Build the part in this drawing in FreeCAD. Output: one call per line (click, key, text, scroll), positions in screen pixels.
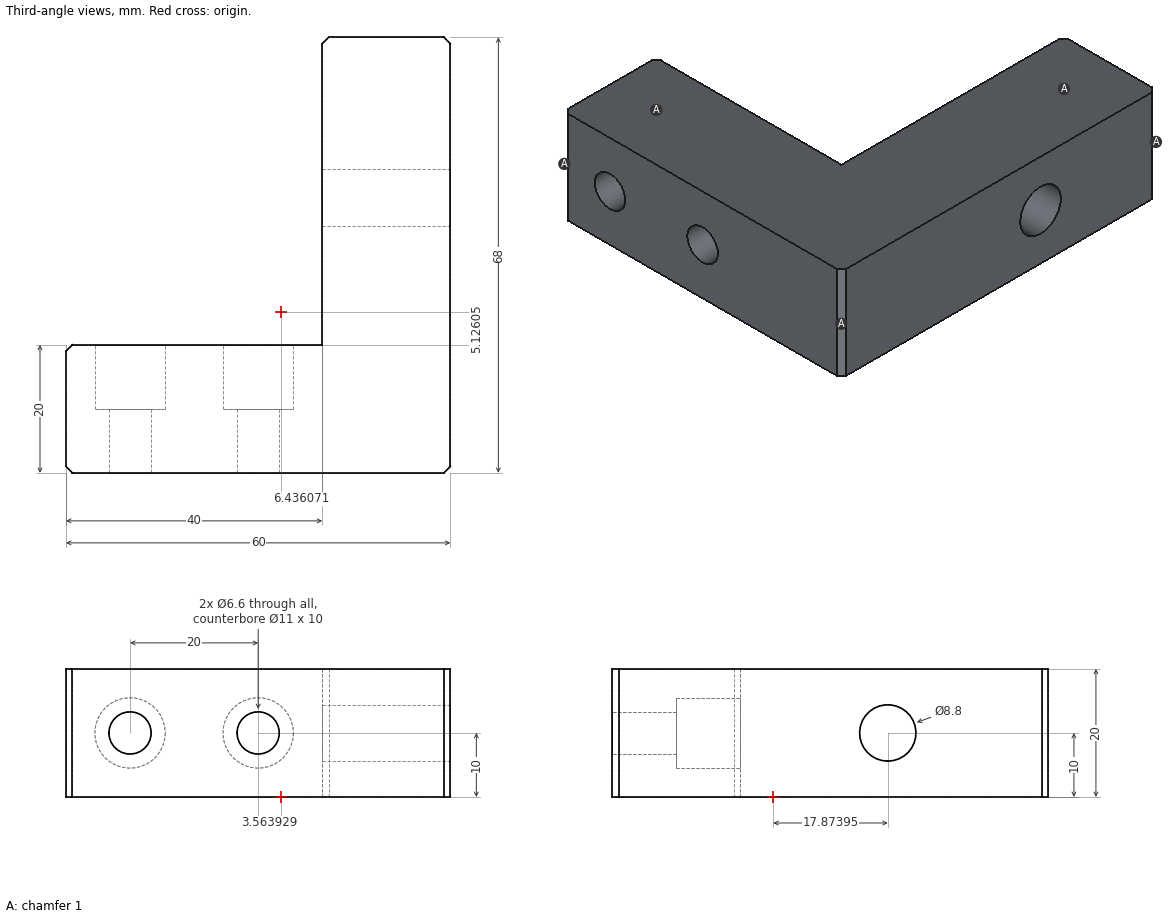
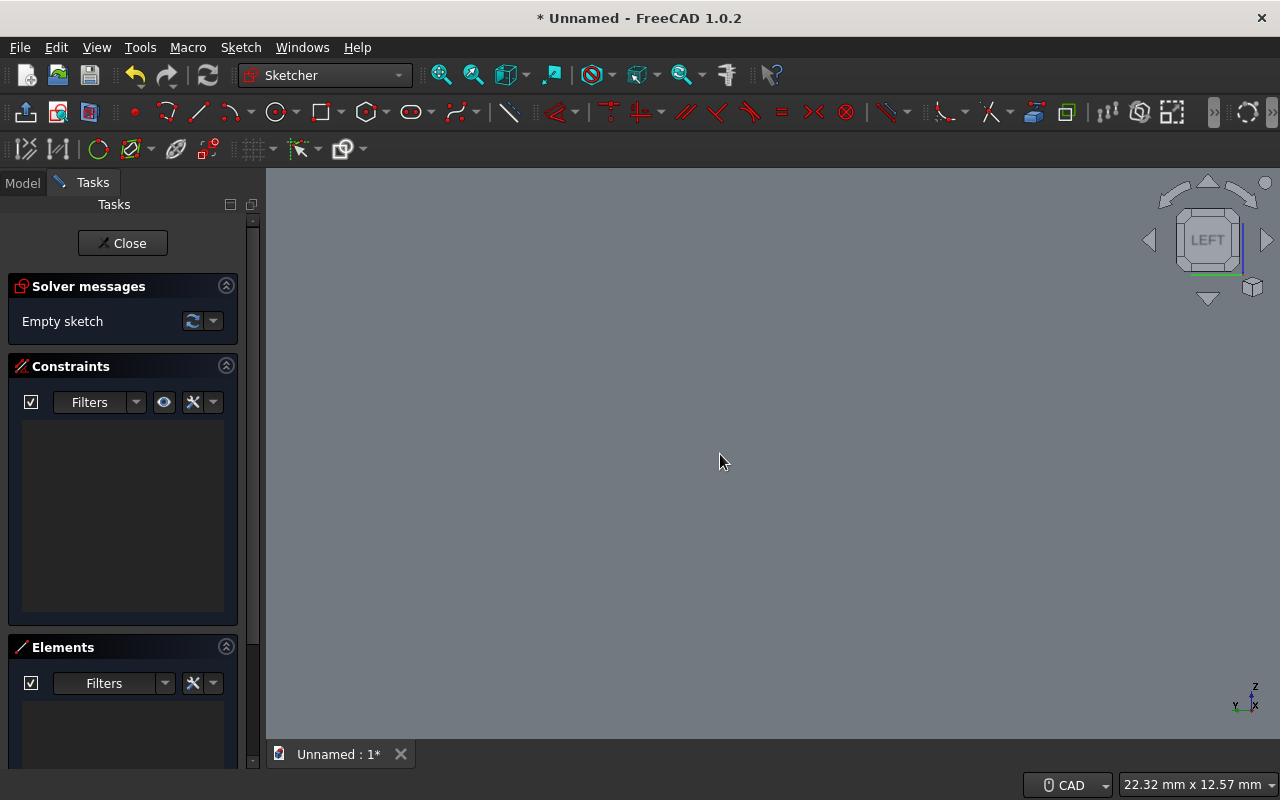
click(276, 112)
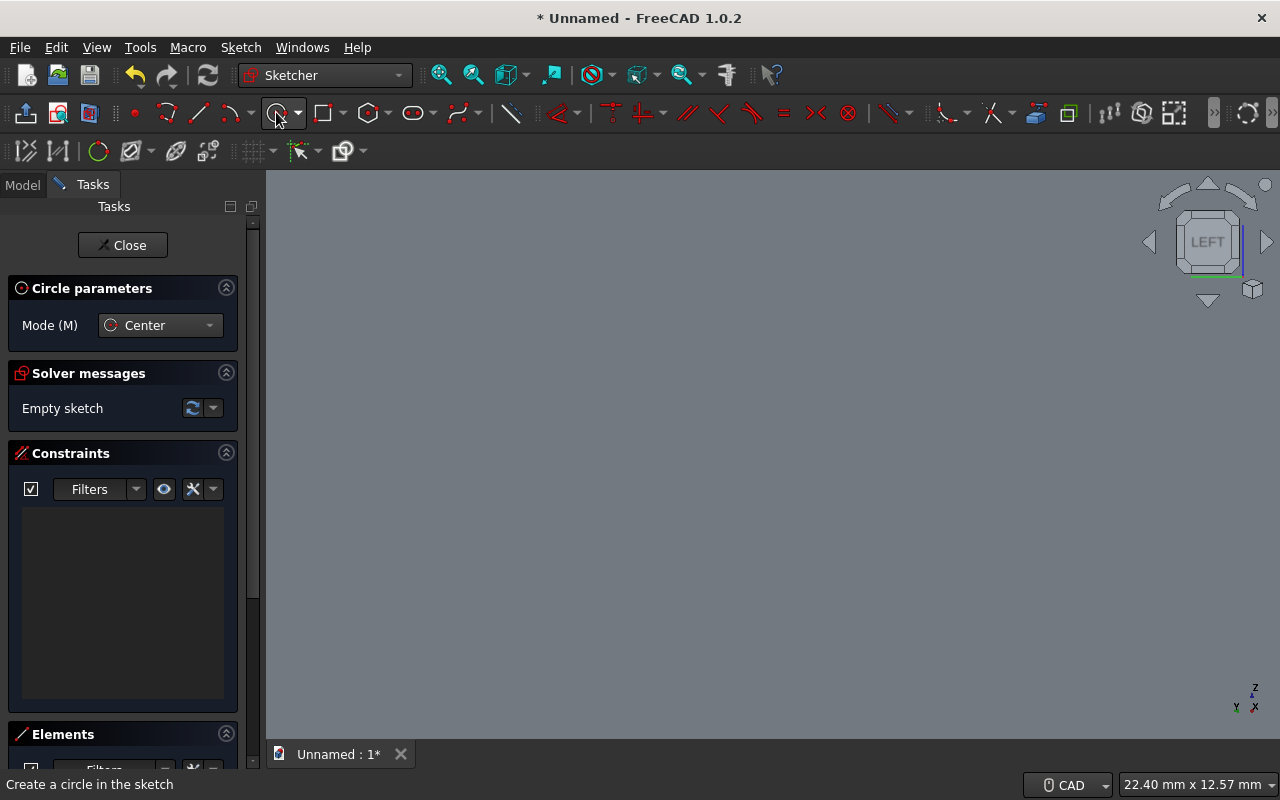
click(700, 448)
move(841, 307)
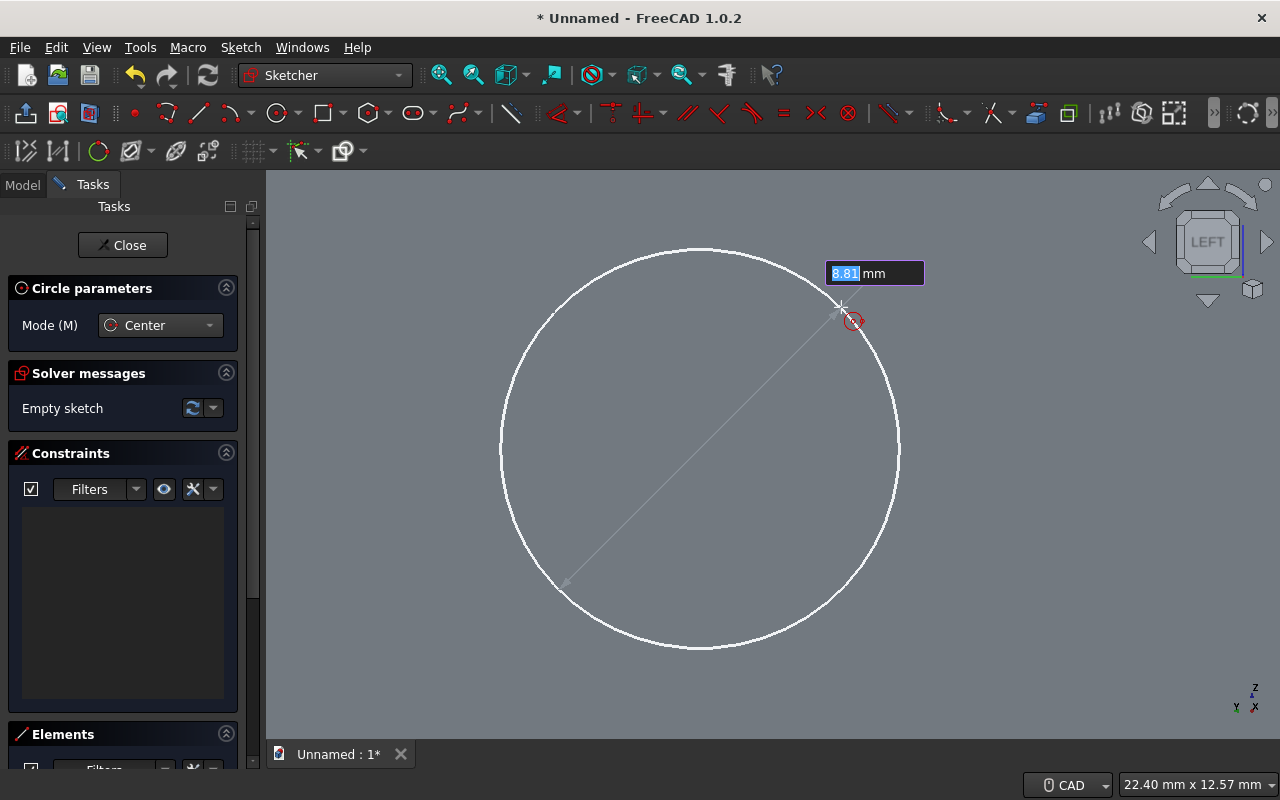
text(8.8)
key(Return)
key(Escape)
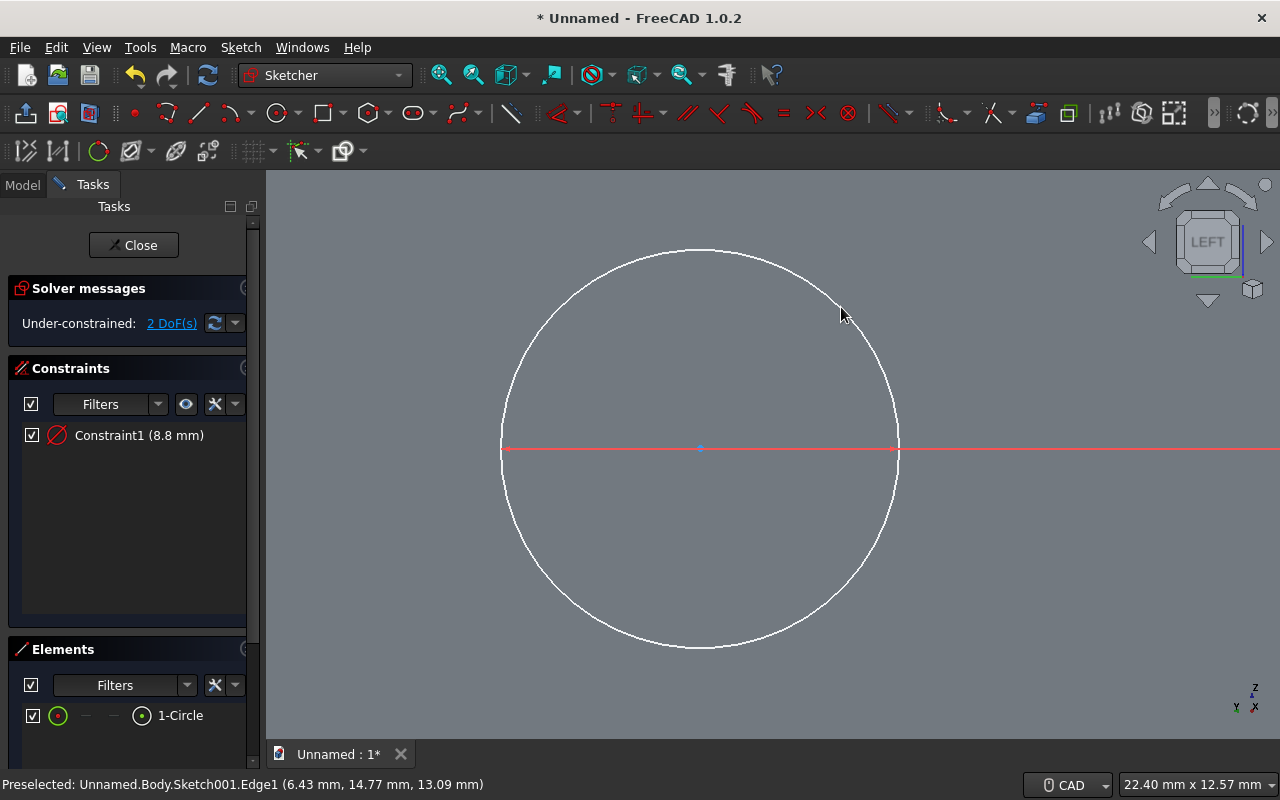
click(558, 114)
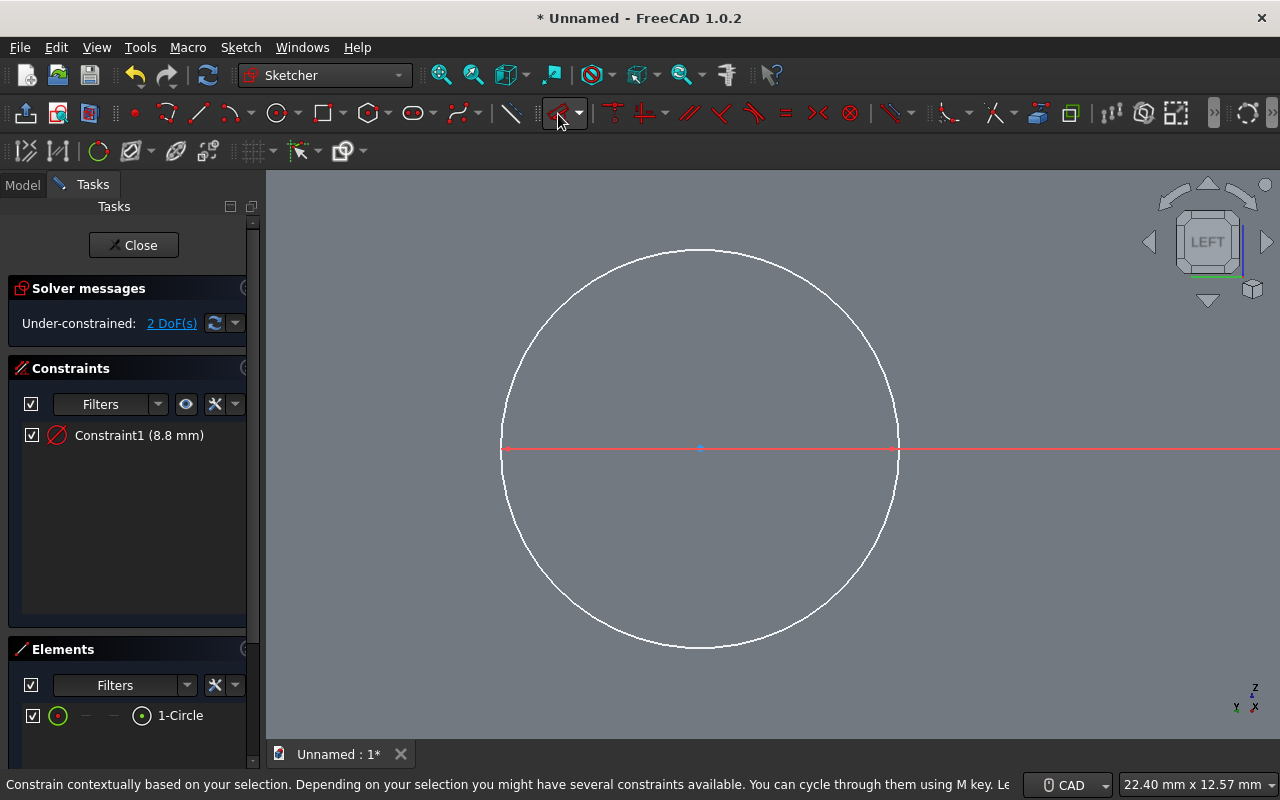
click(700, 449)
click(666, 580)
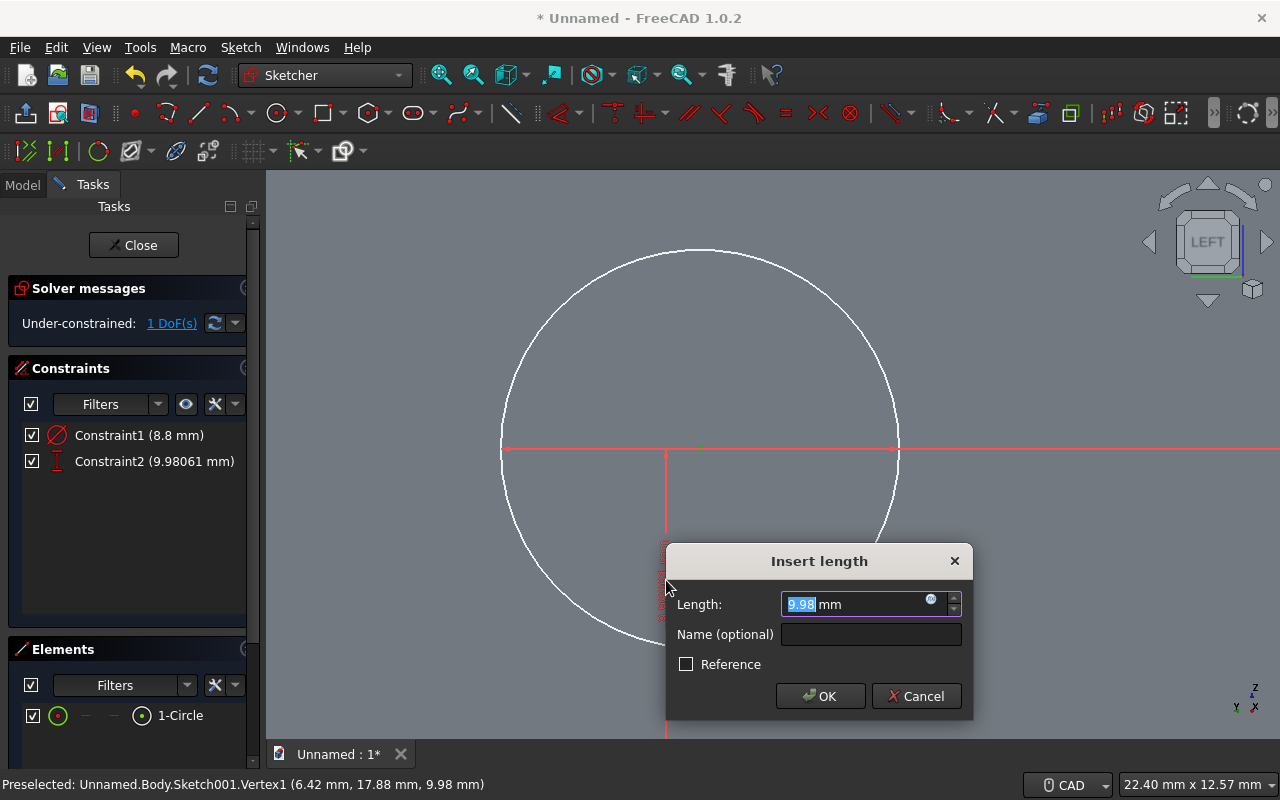
text(10)
key(Return)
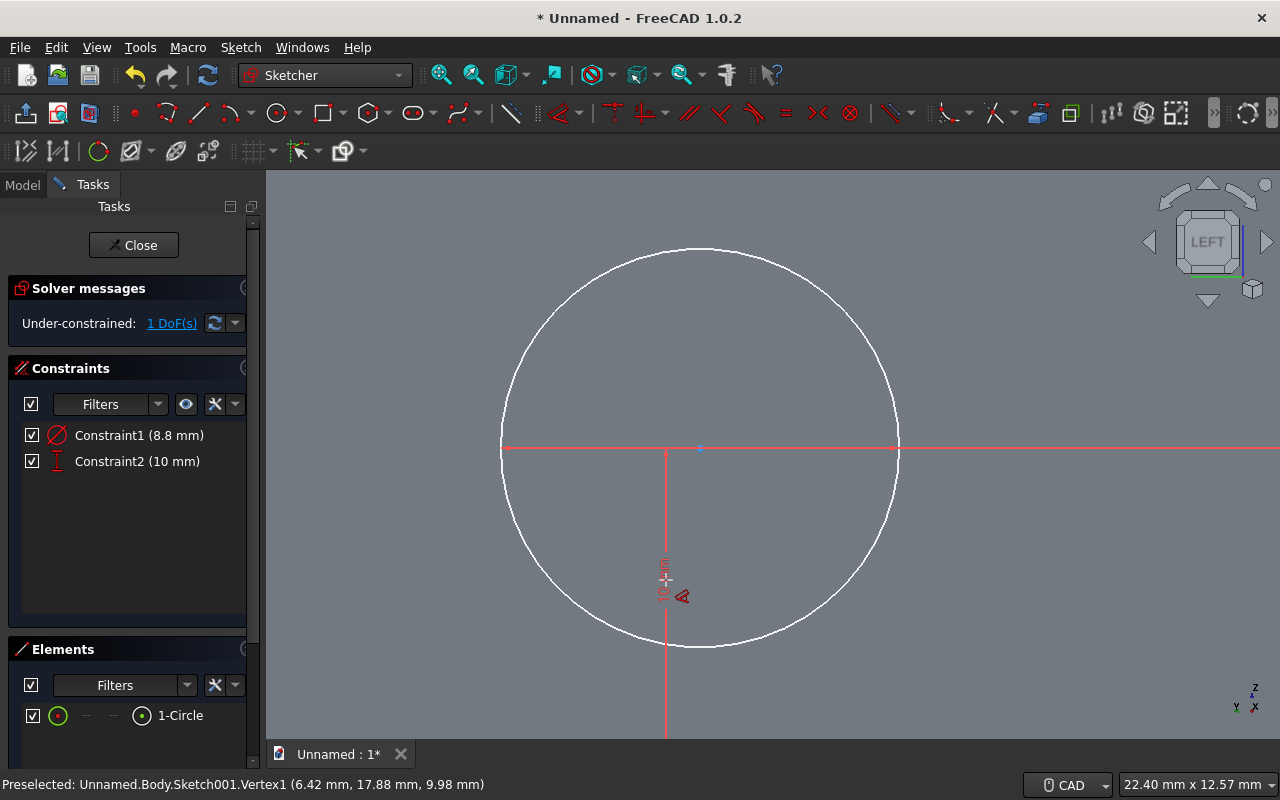
click(700, 448)
click(812, 414)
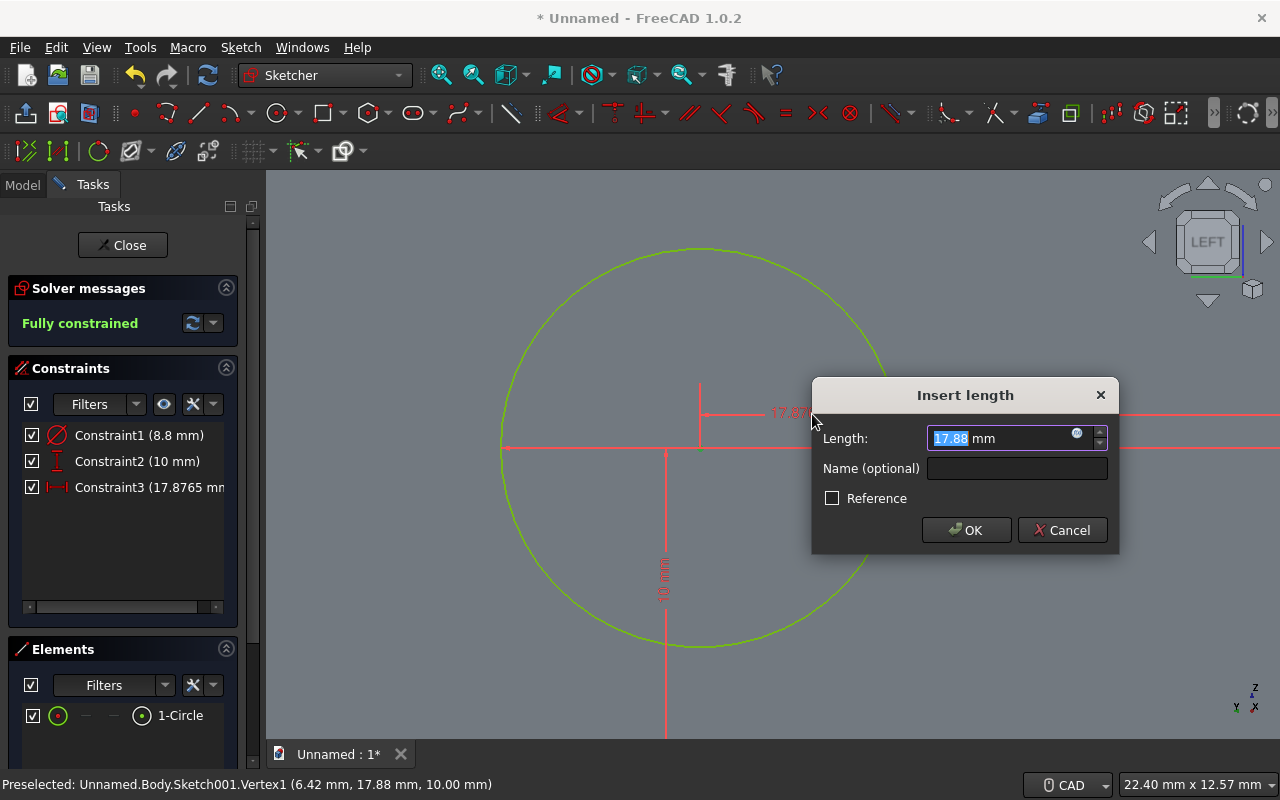
text(17.87395)
key(Return)
key(Escape)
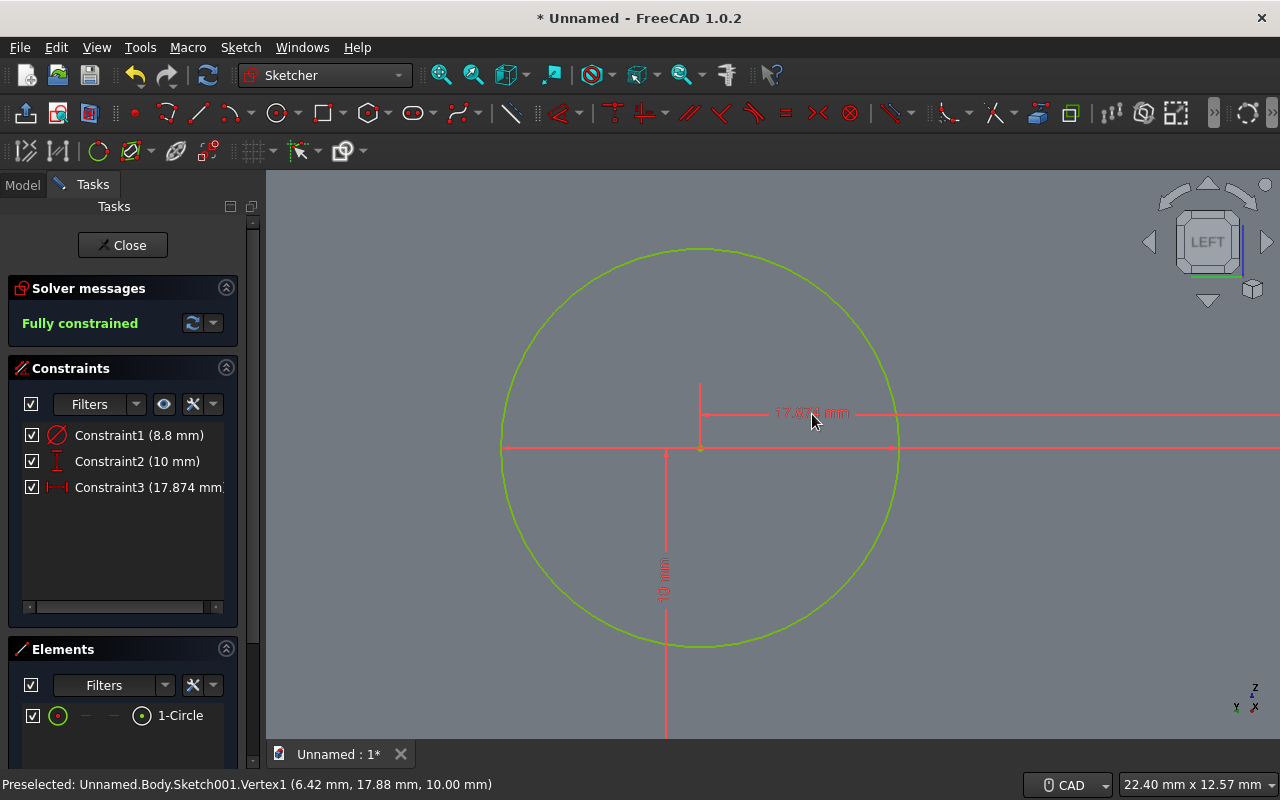
click(123, 245)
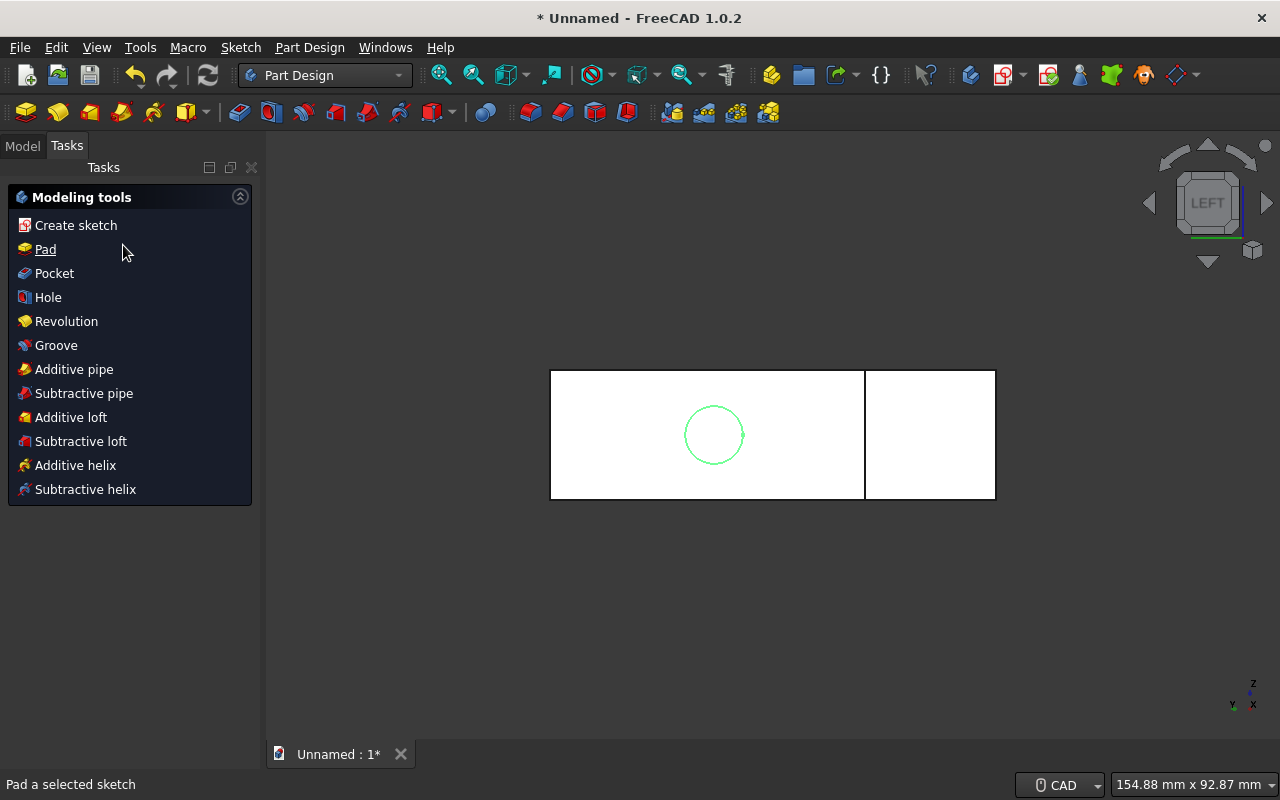
click(240, 112)